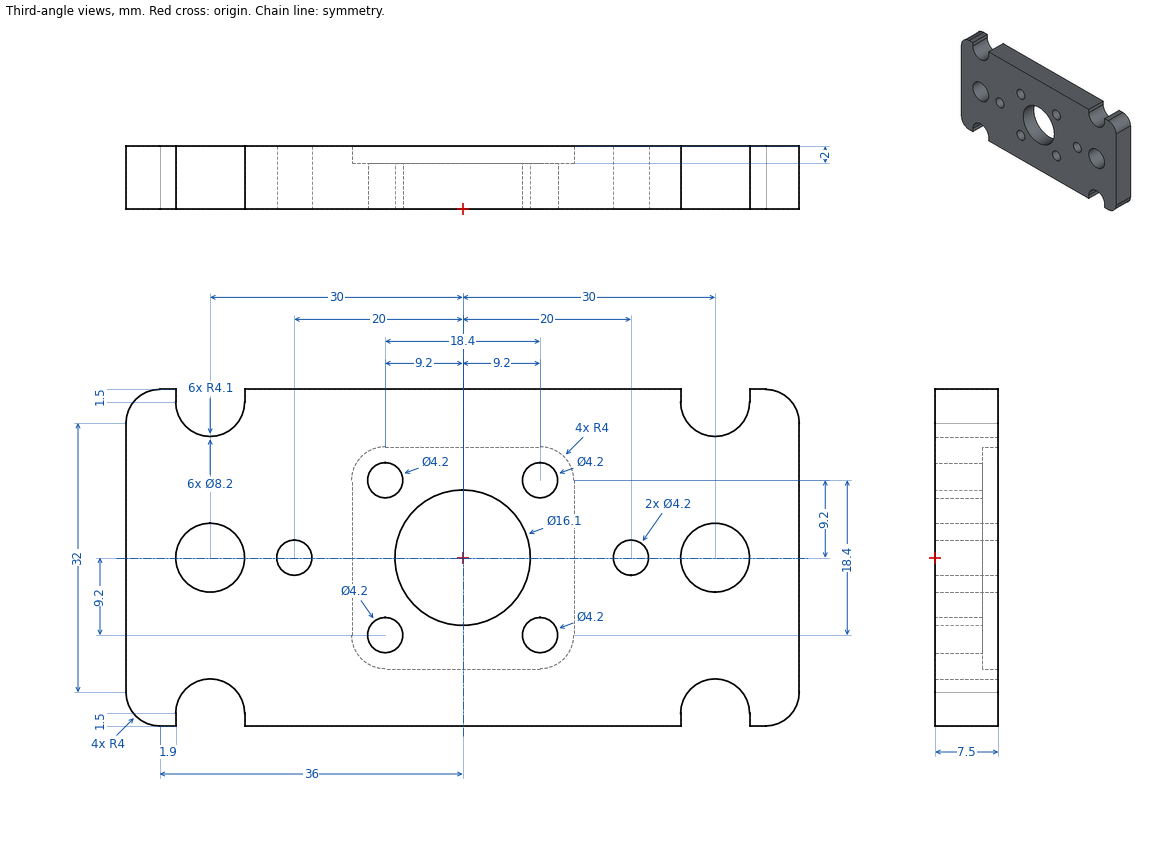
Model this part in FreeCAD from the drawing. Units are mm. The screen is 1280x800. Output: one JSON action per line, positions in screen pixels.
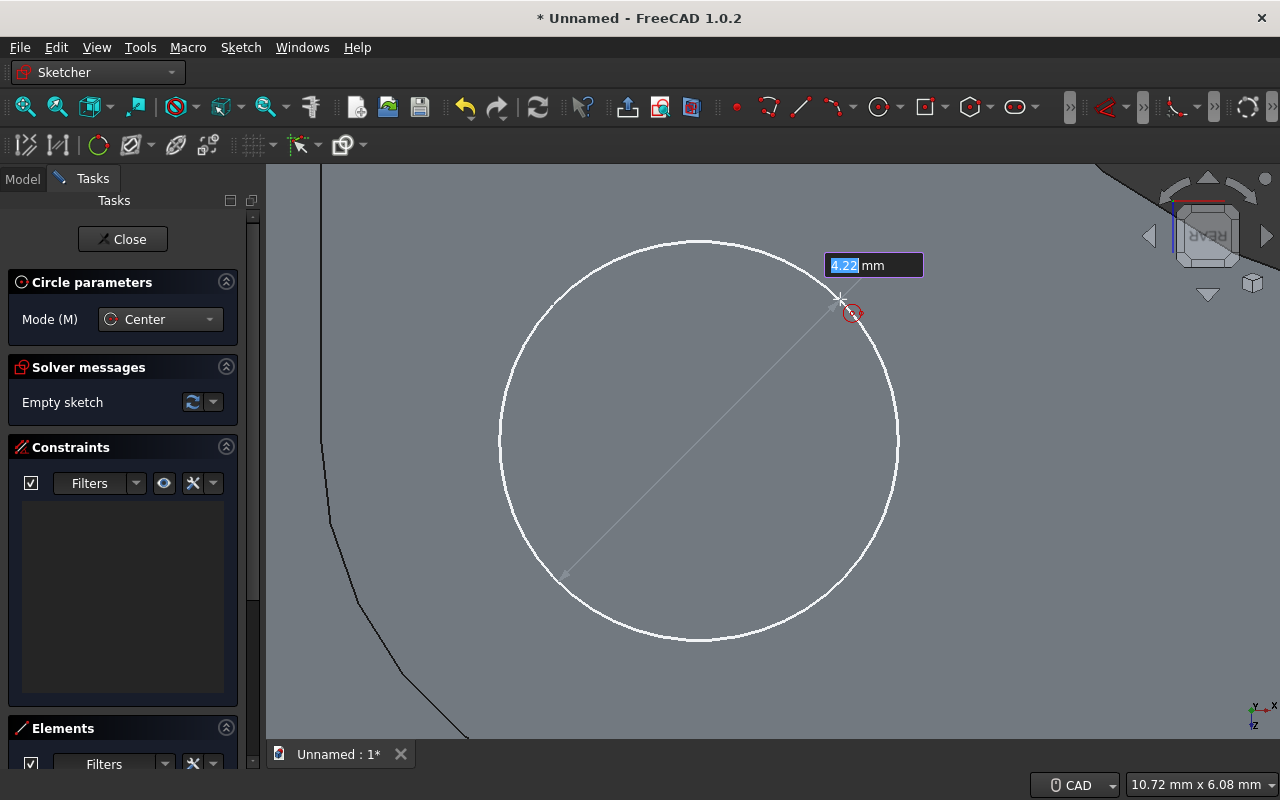
{"action": "type", "text": "4.2"}
{"action": "key", "text": "Return"}
{"action": "key", "text": "Escape"}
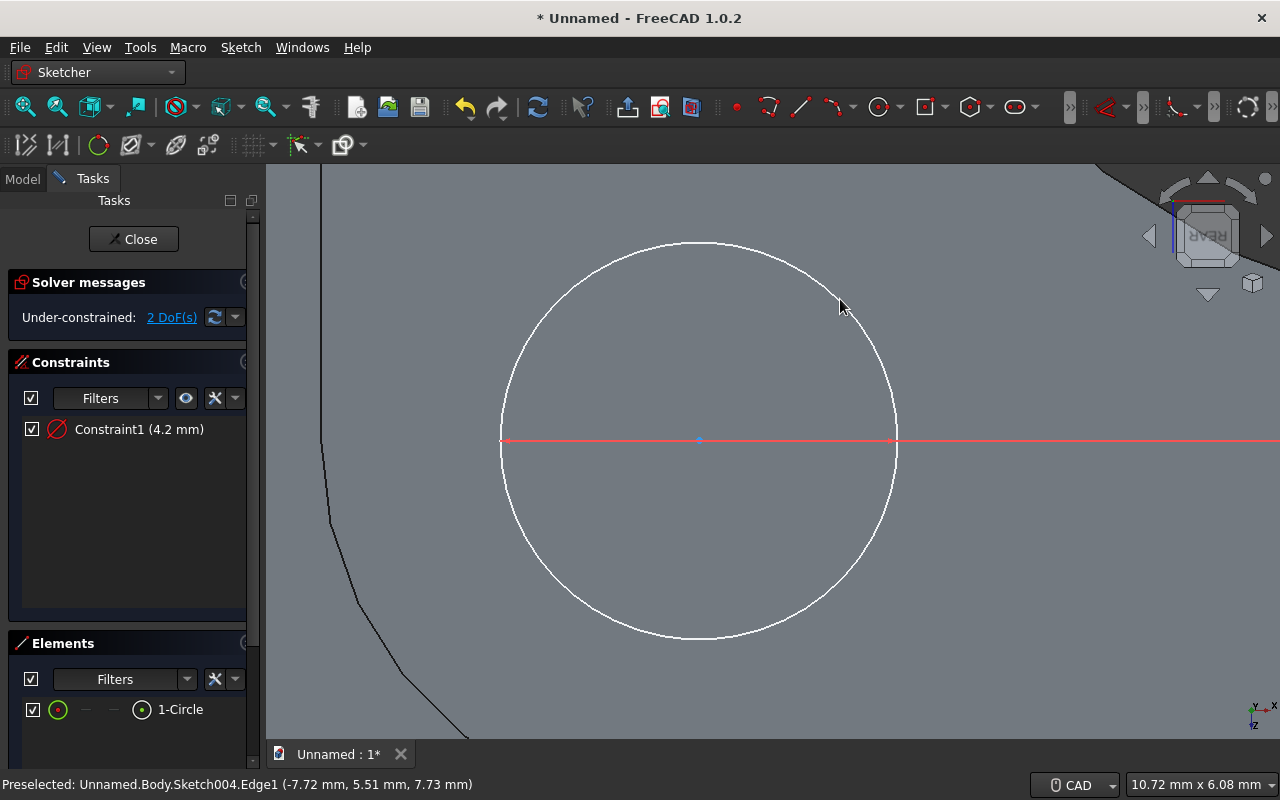
{"action": "left_click", "coordinate": [1106, 108]}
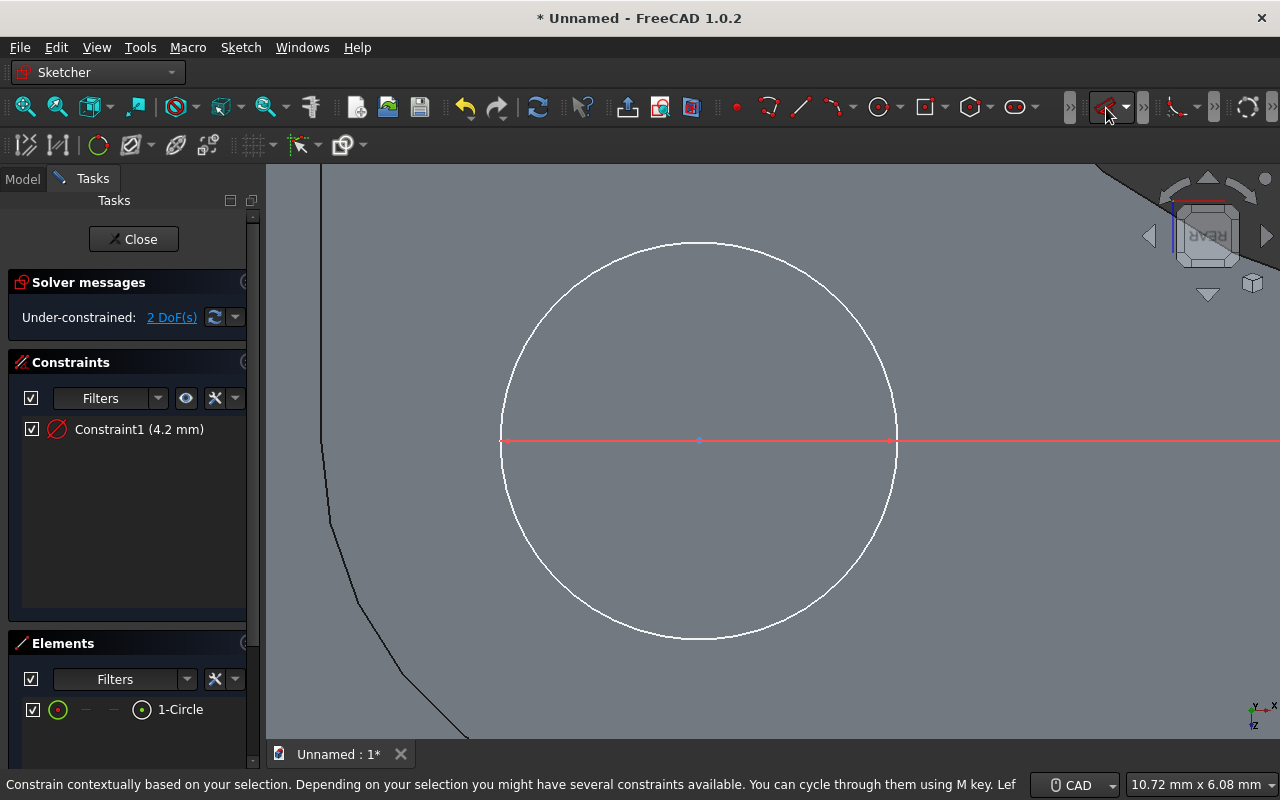
{"action": "left_click", "coordinate": [699, 441]}
{"action": "left_click", "coordinate": [811, 475]}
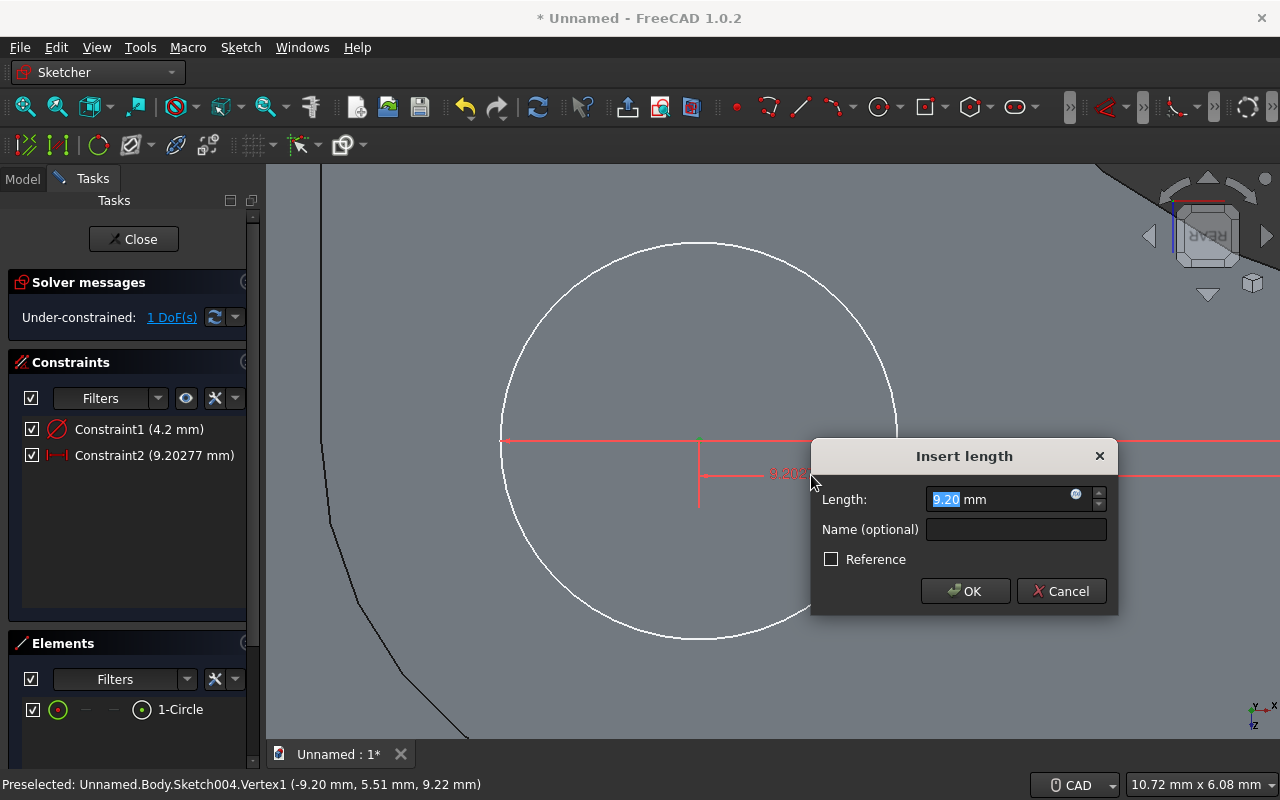
{"action": "type", "text": "9.2"}
{"action": "key", "text": "Return"}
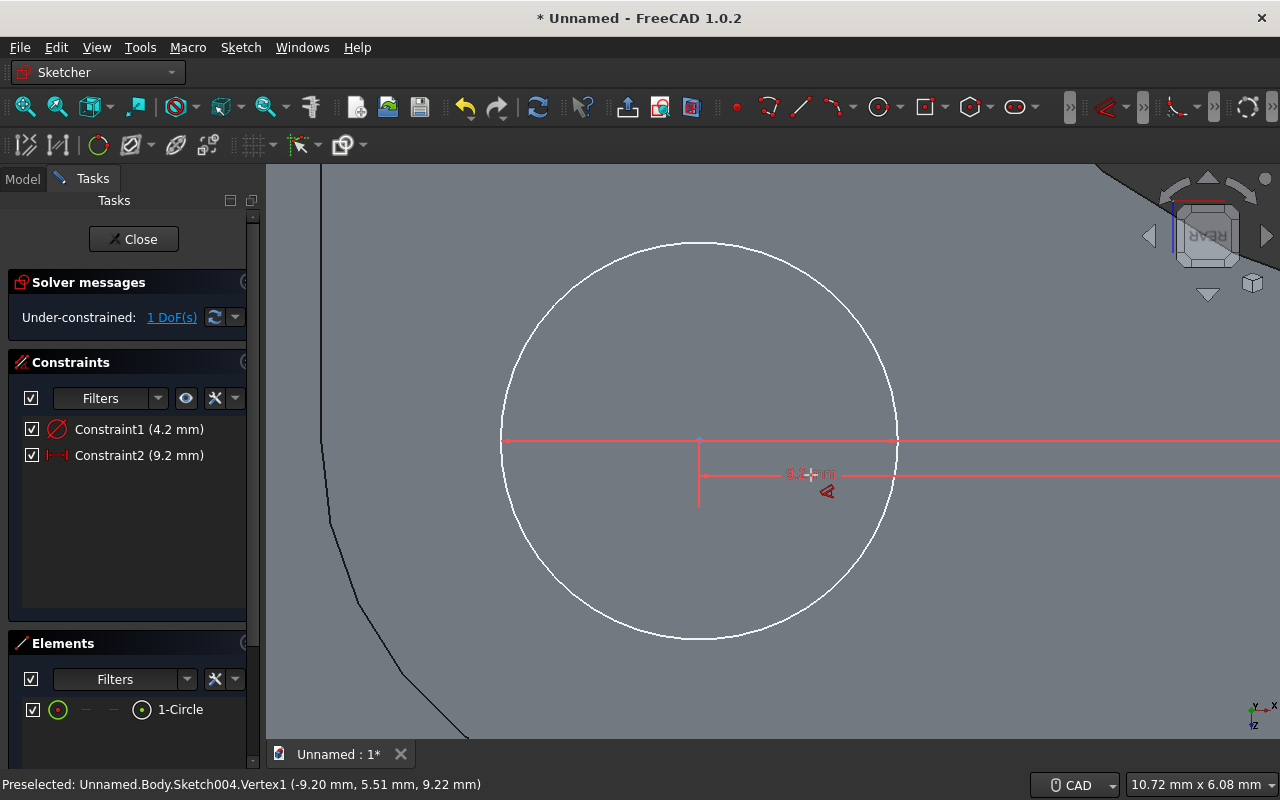
{"action": "left_click", "coordinate": [699, 441]}
{"action": "left_click", "coordinate": [665, 316]}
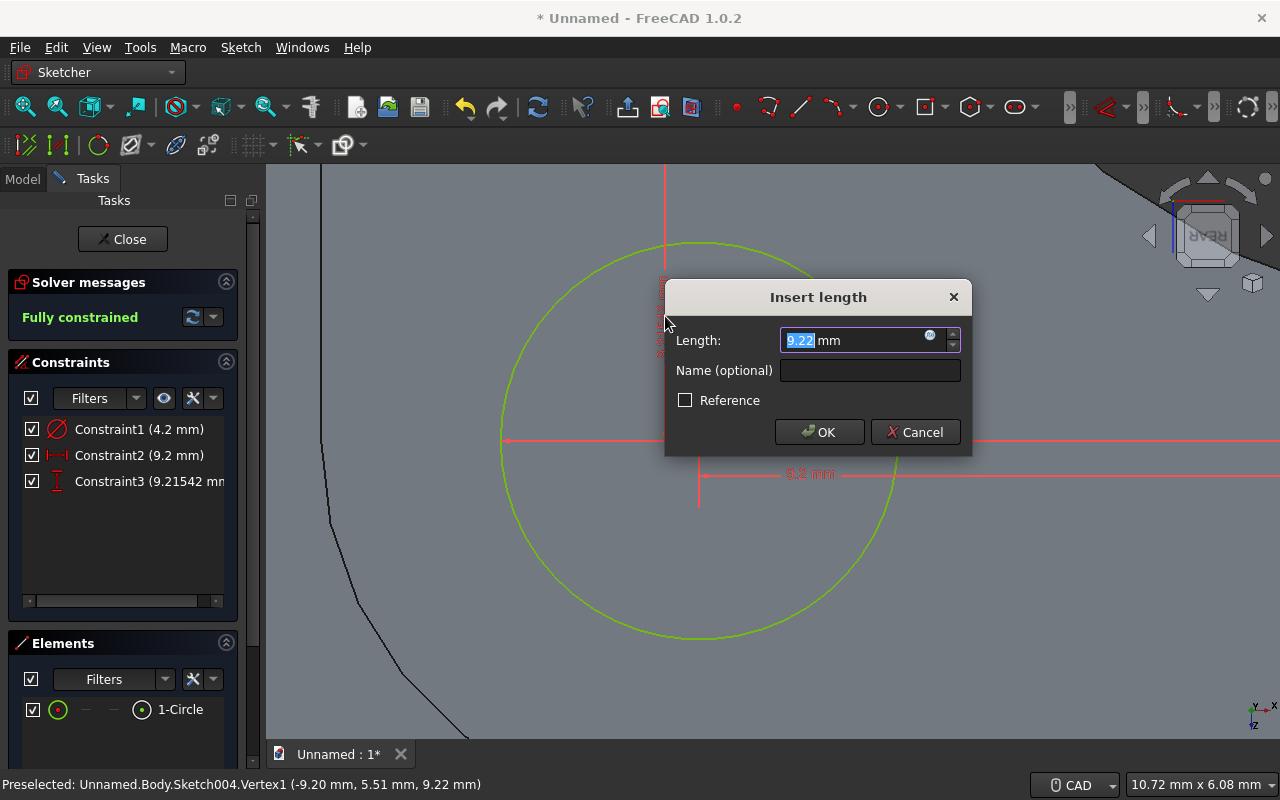
{"action": "type", "text": "9.2"}
{"action": "key", "text": "Return"}
{"action": "key", "text": "Escape"}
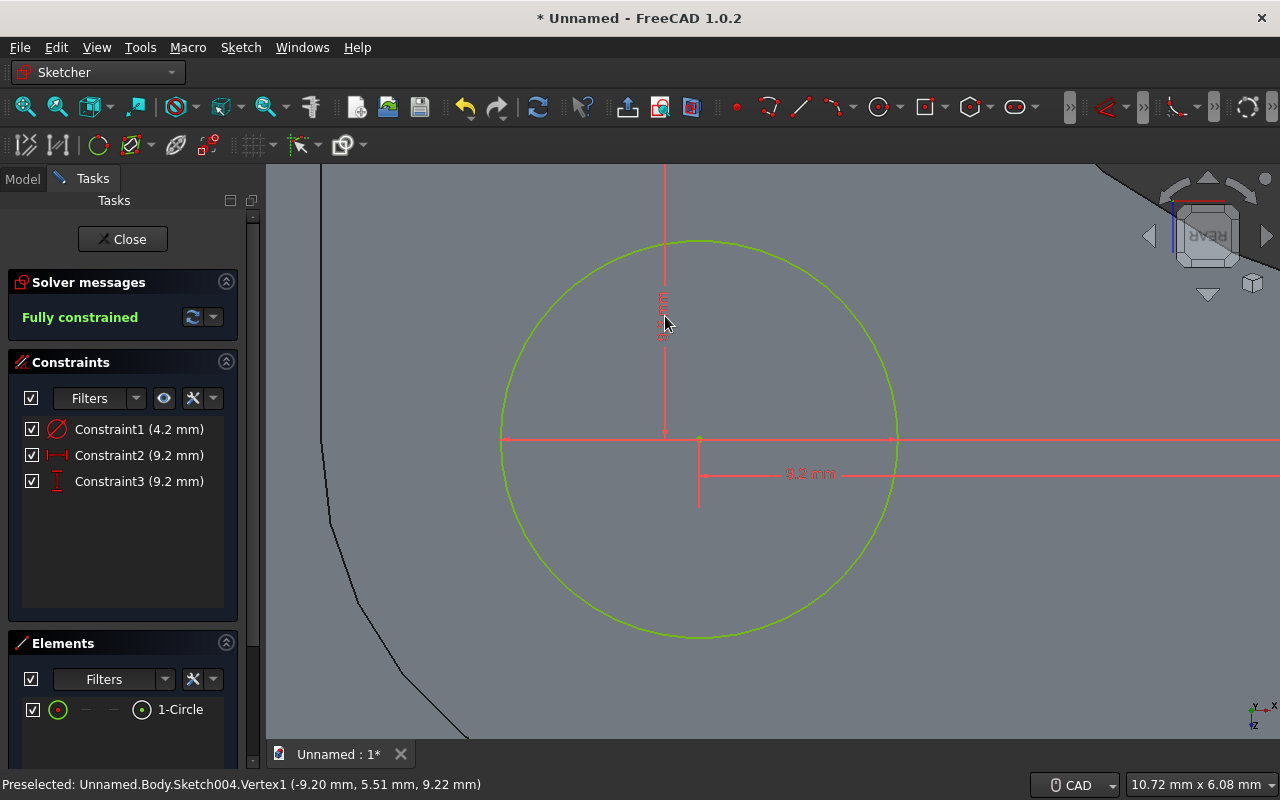
{"action": "left_click", "coordinate": [123, 239]}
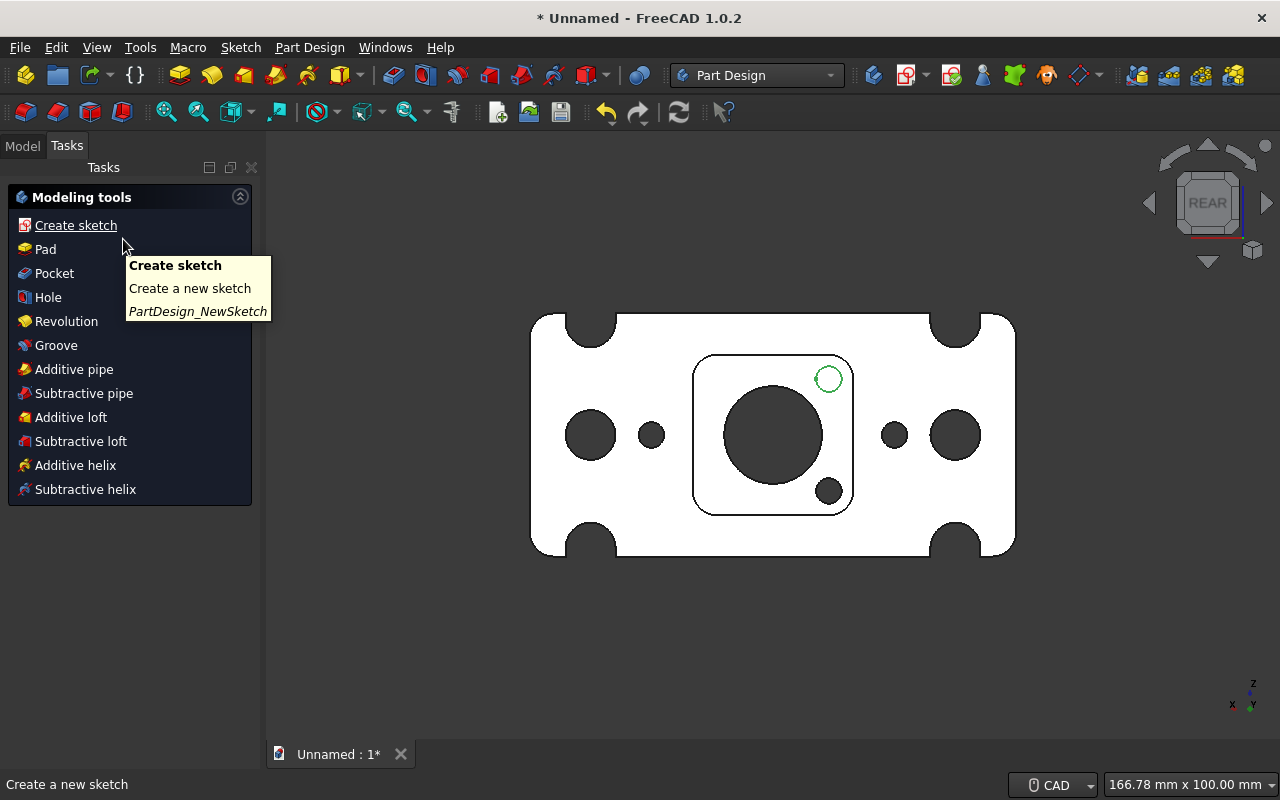
{"action": "left_click", "coordinate": [394, 76]}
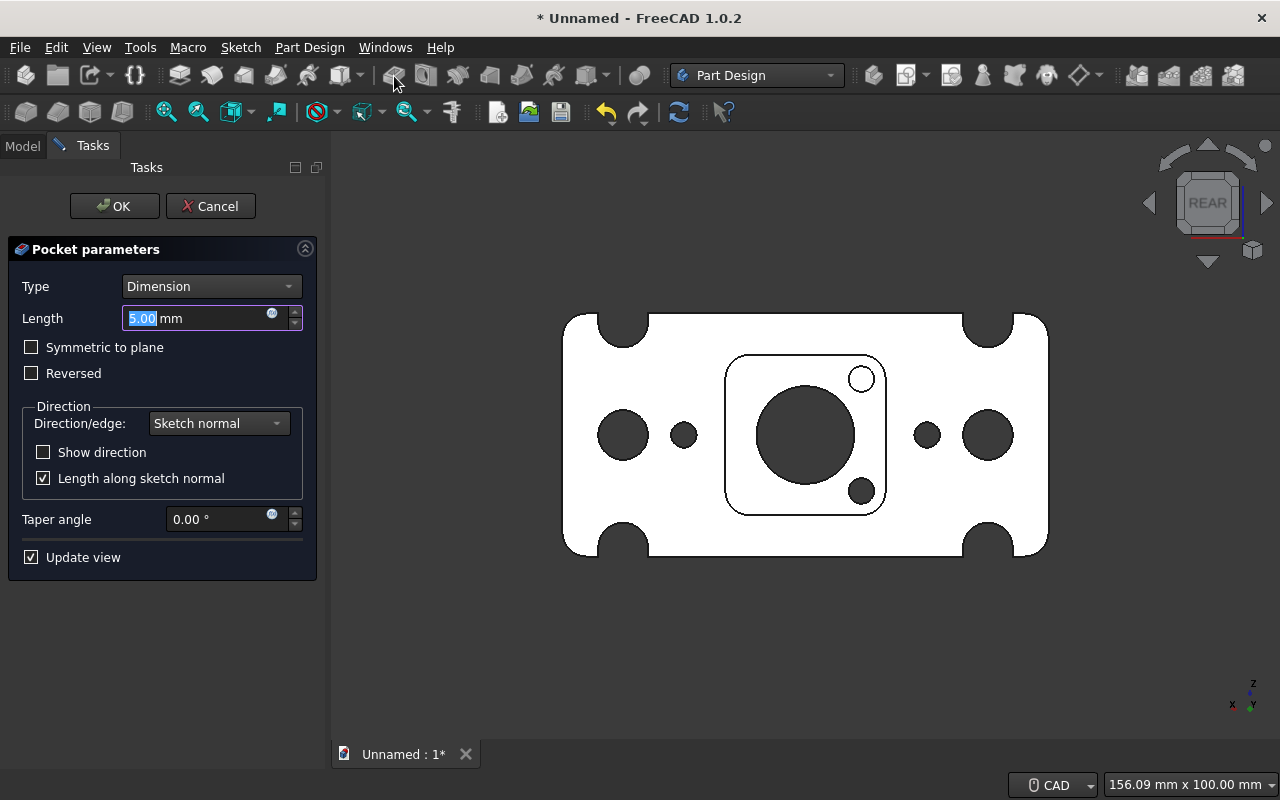
{"action": "left_click", "coordinate": [212, 286]}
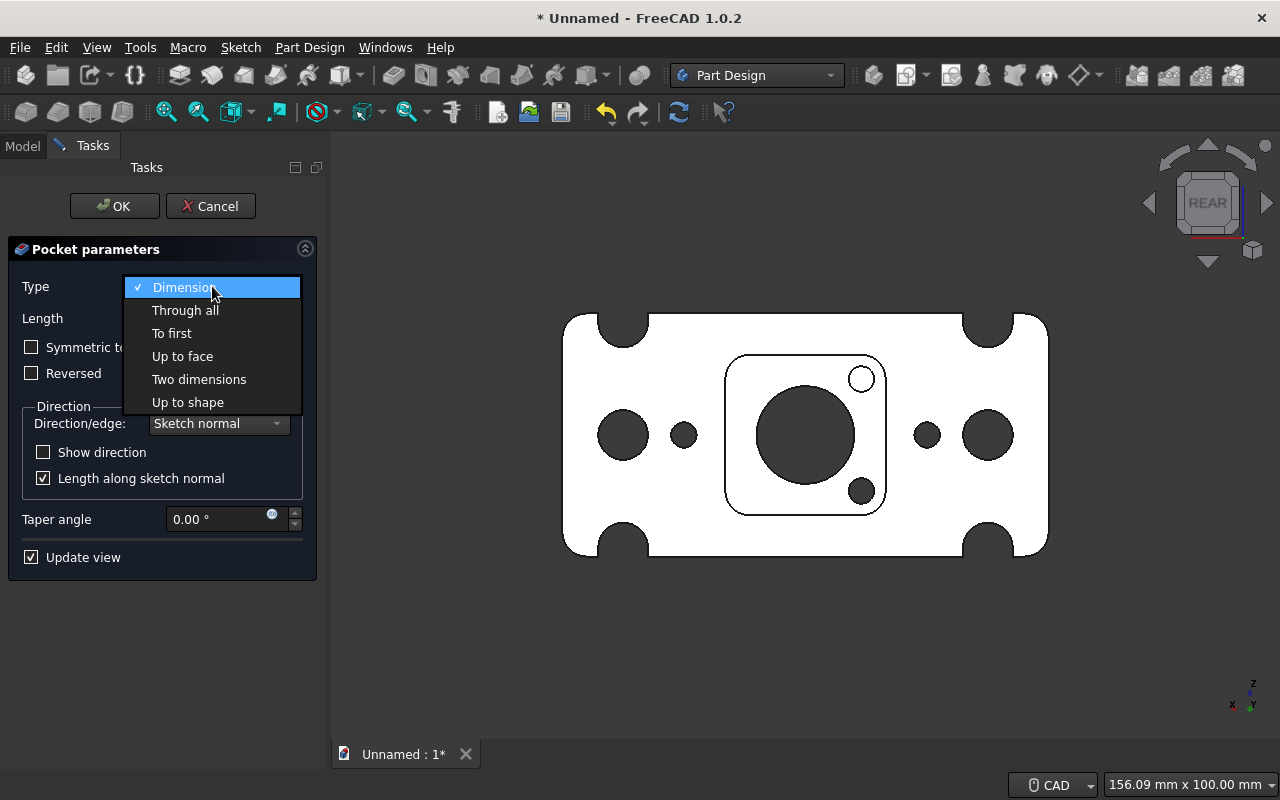
{"action": "left_click", "coordinate": [212, 334]}